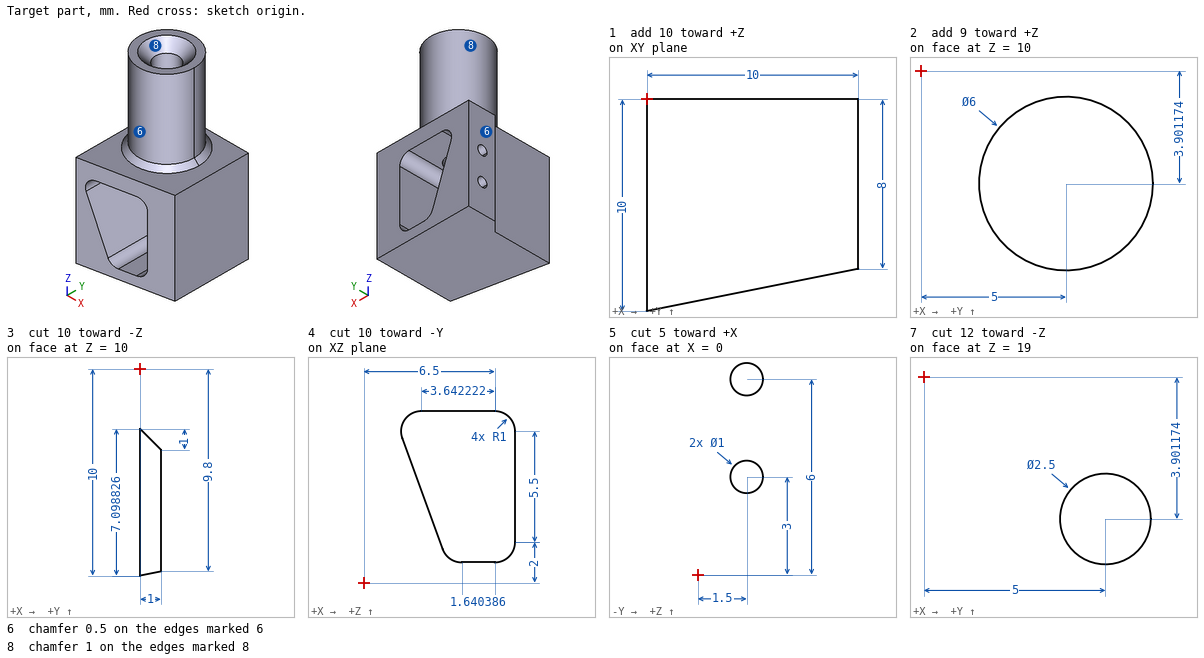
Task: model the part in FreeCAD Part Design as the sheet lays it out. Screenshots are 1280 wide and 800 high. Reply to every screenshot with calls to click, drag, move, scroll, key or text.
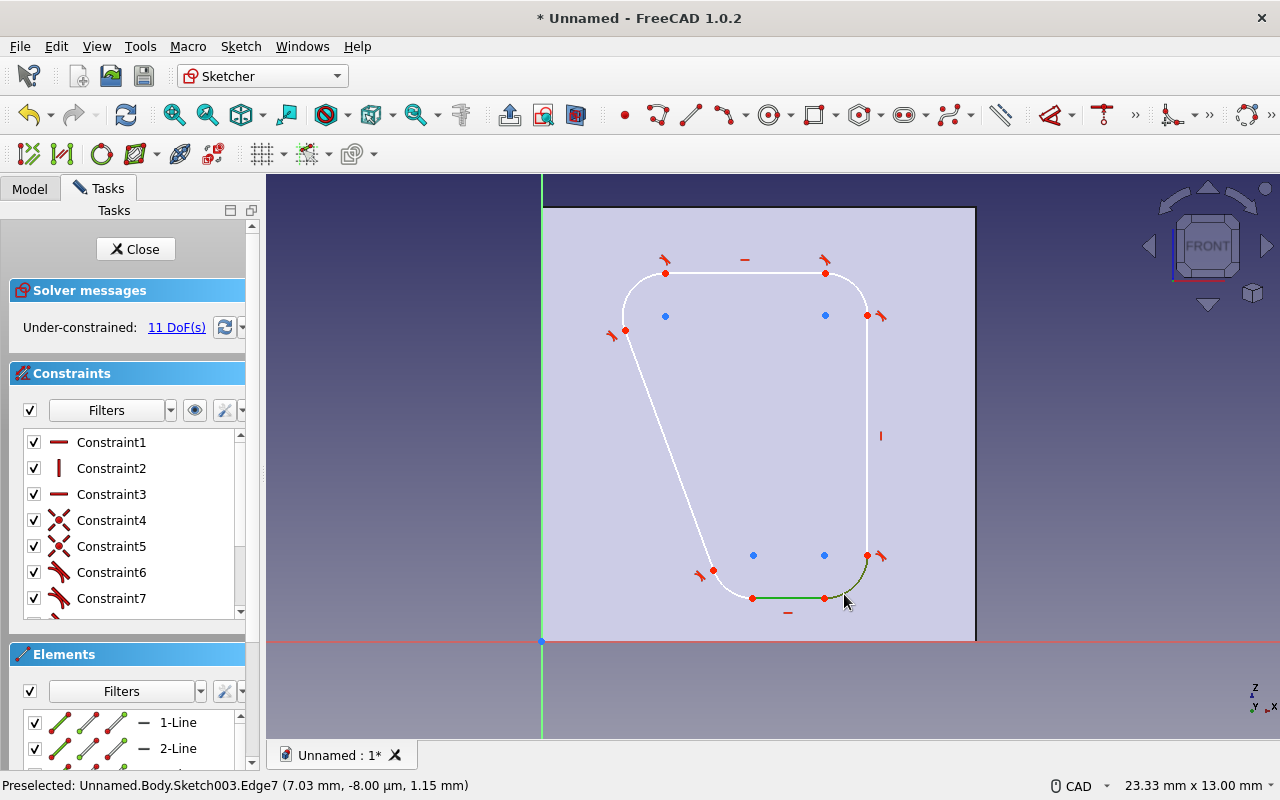
key(t)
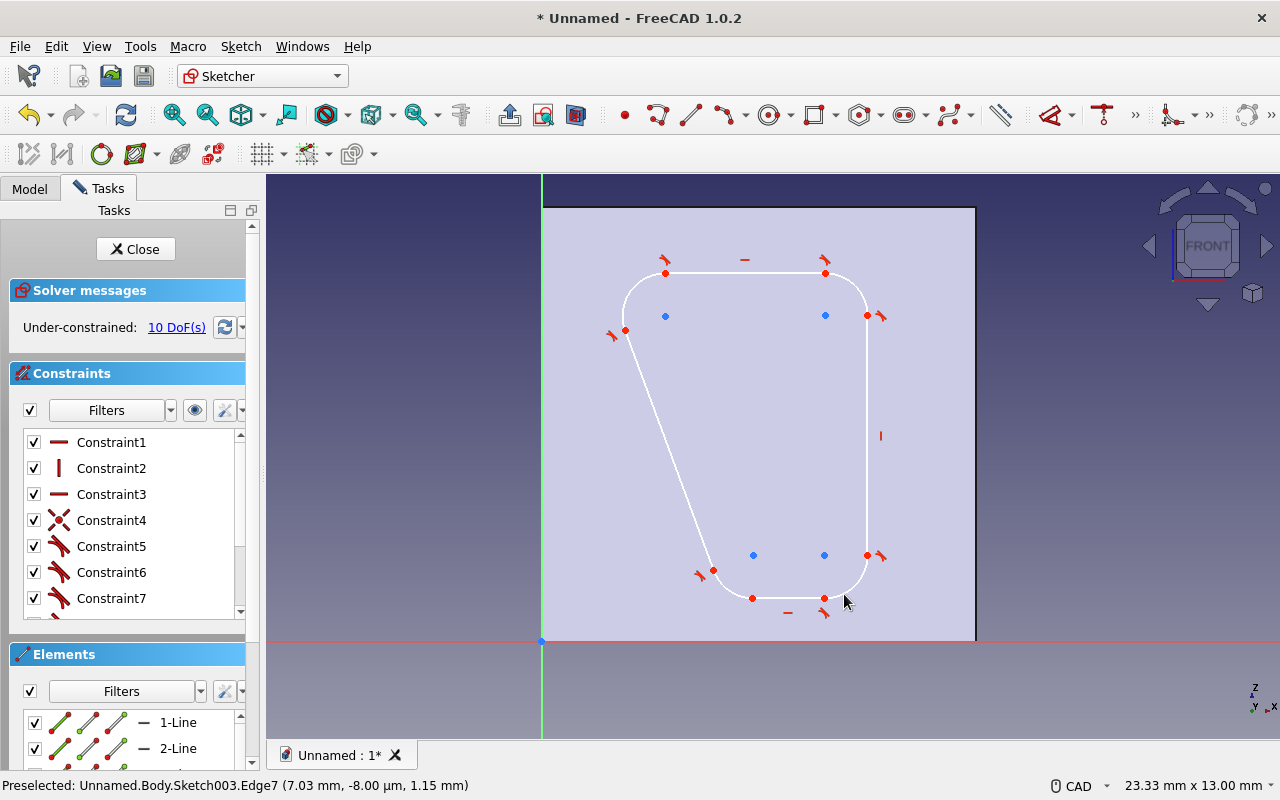
click(803, 598)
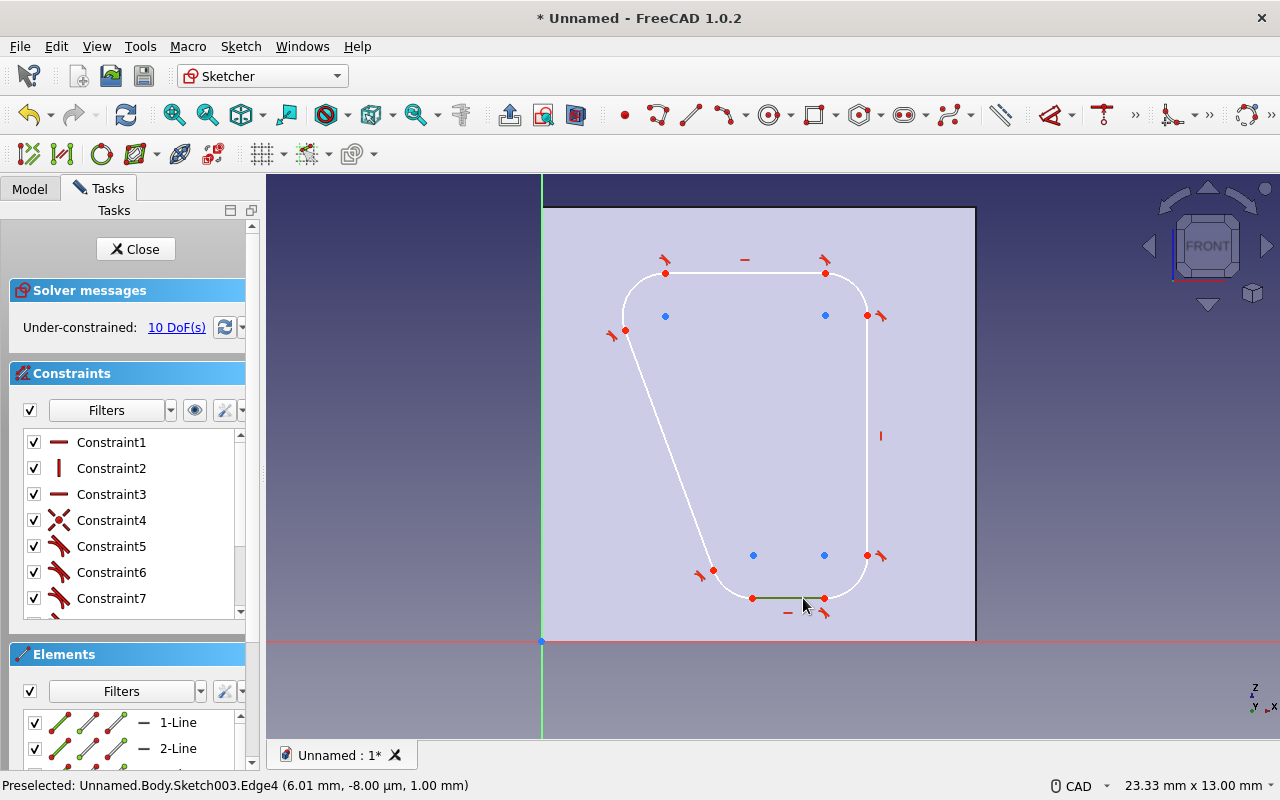
click(721, 583)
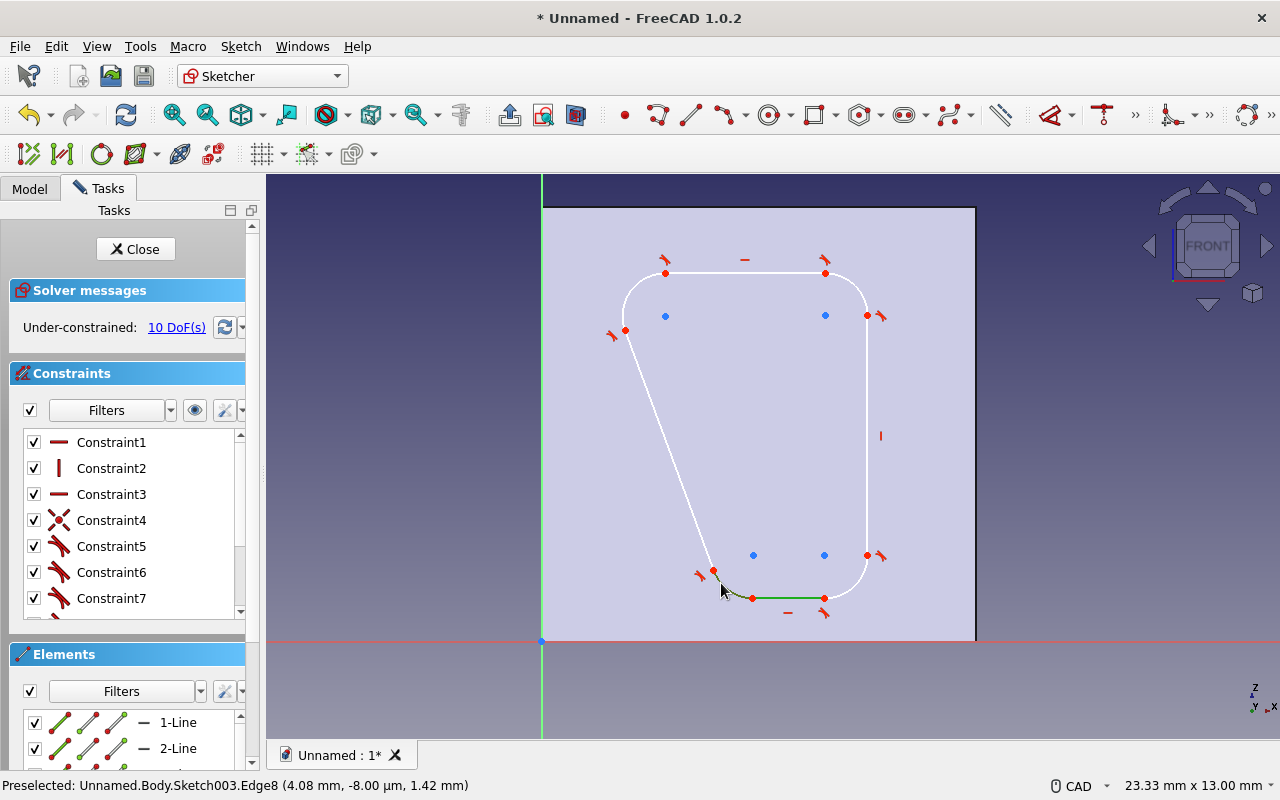
key(t)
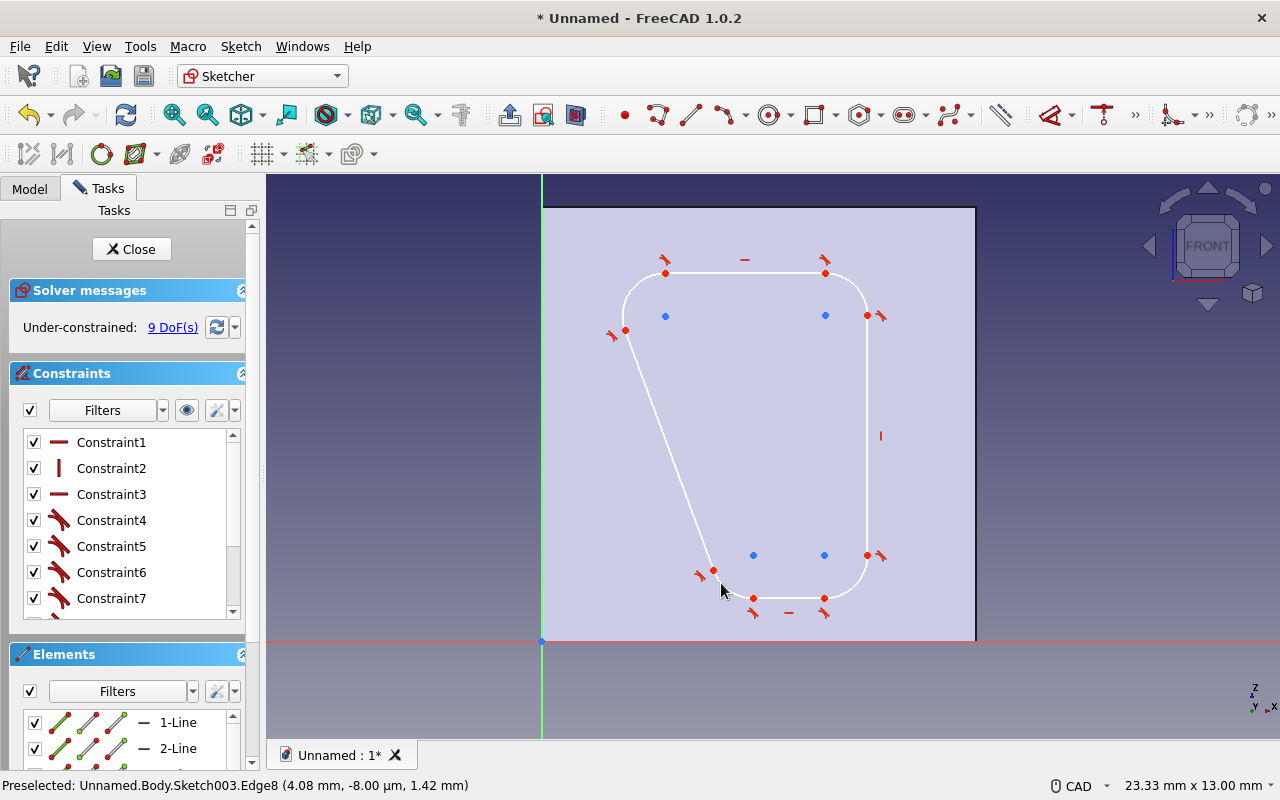
click(642, 280)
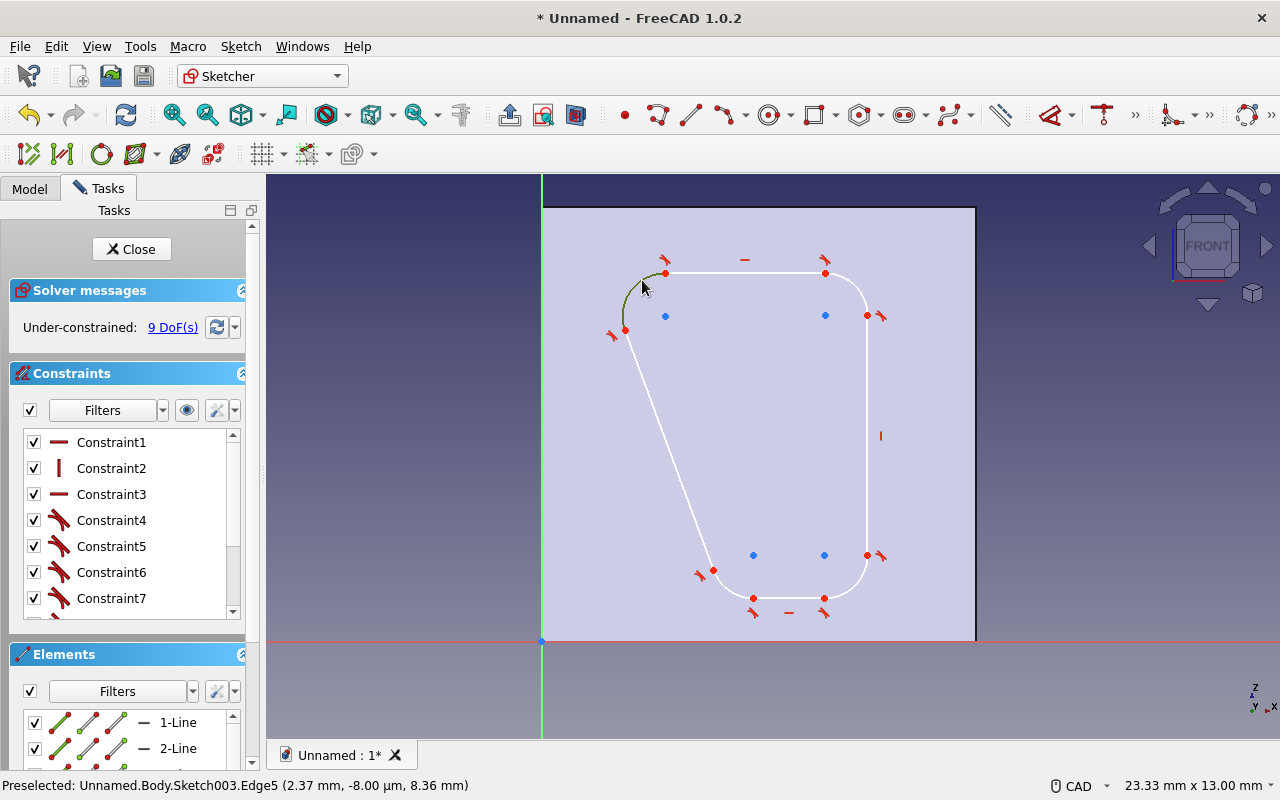
click(863, 296)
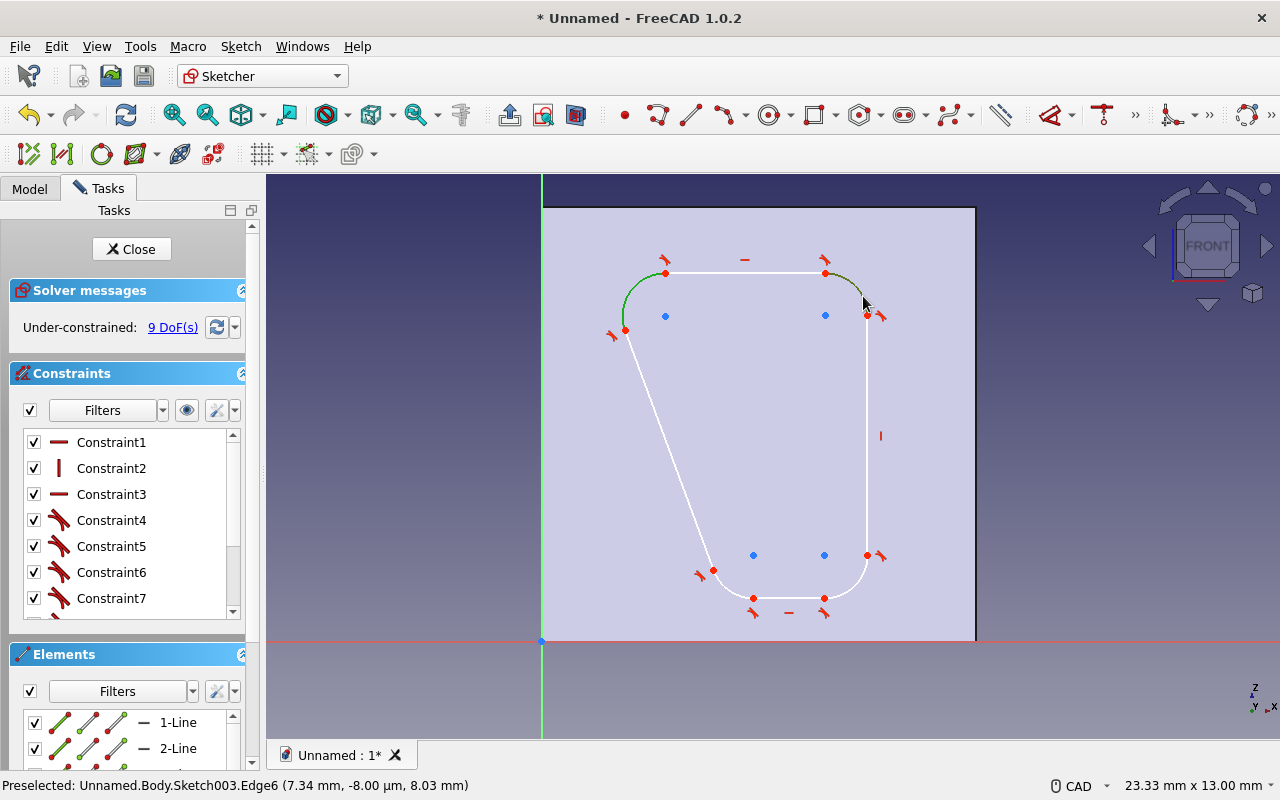
click(844, 594)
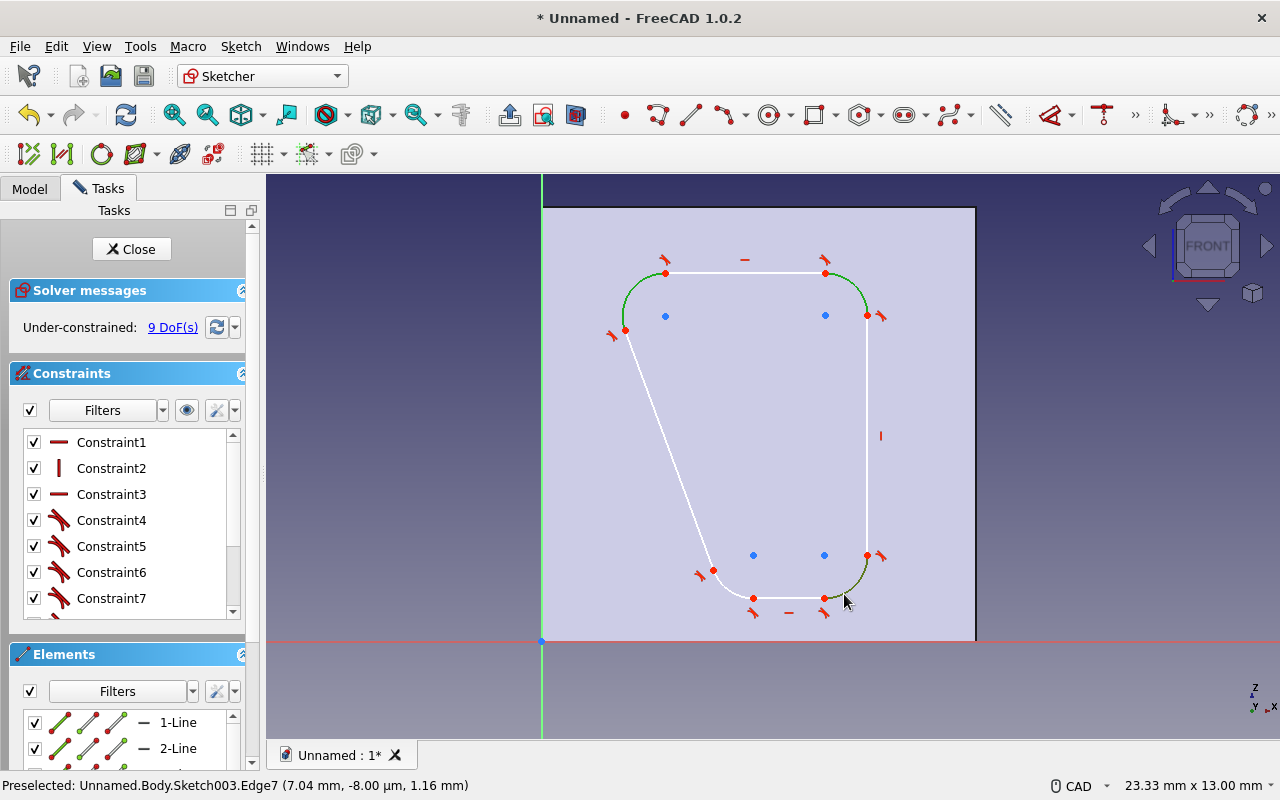
click(722, 584)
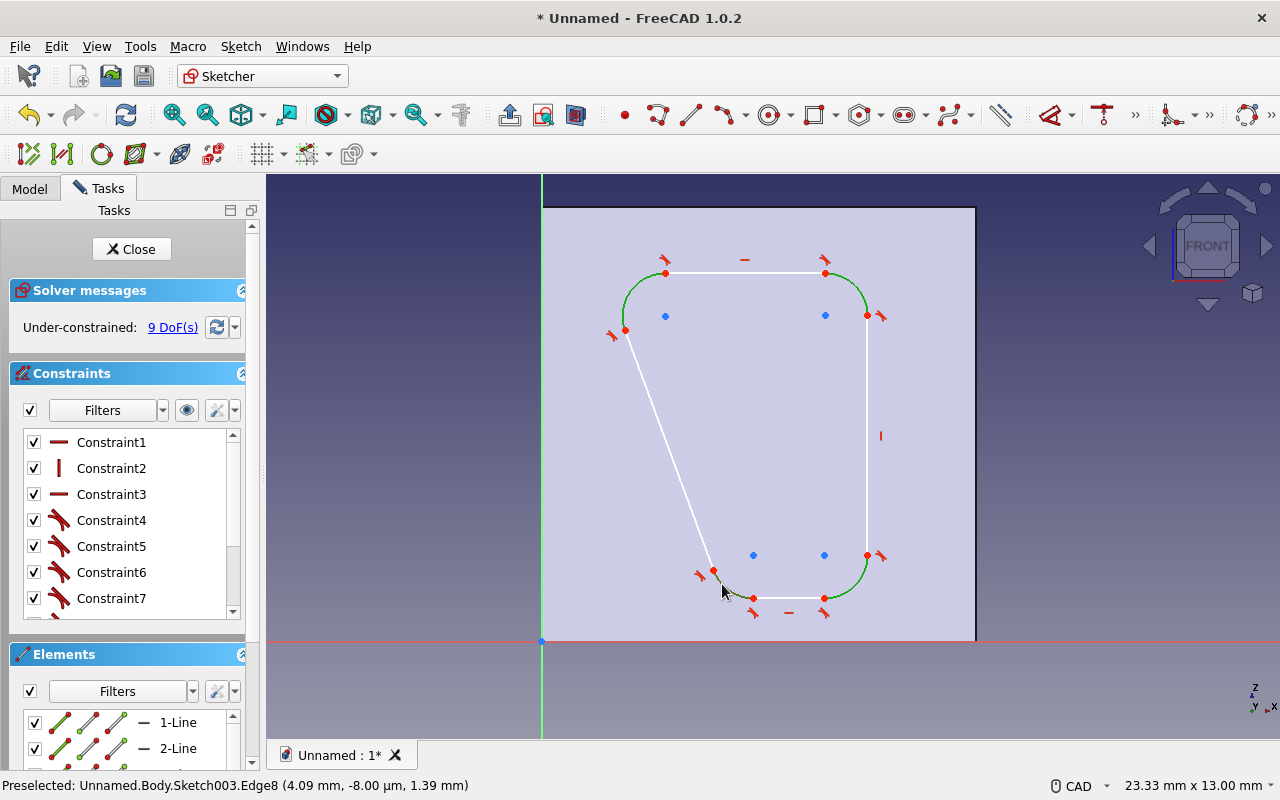
key(e)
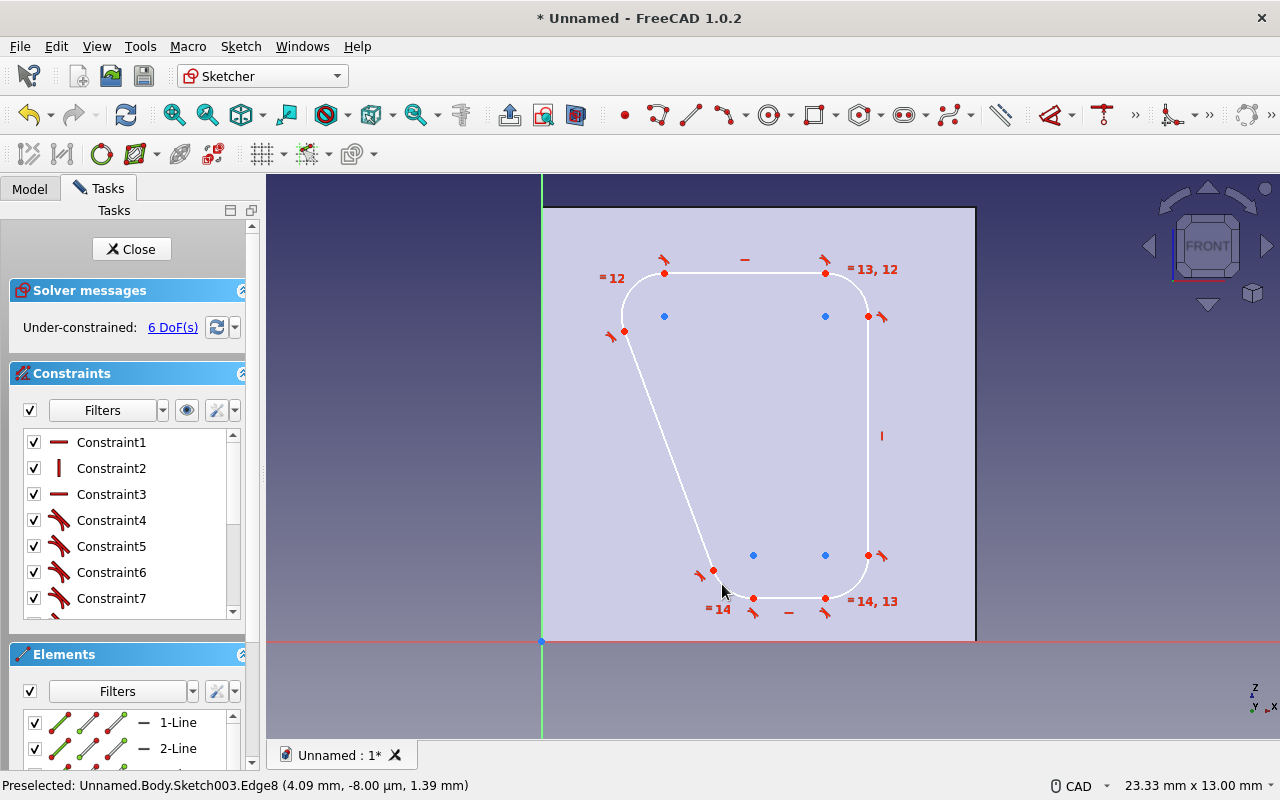
key(d)